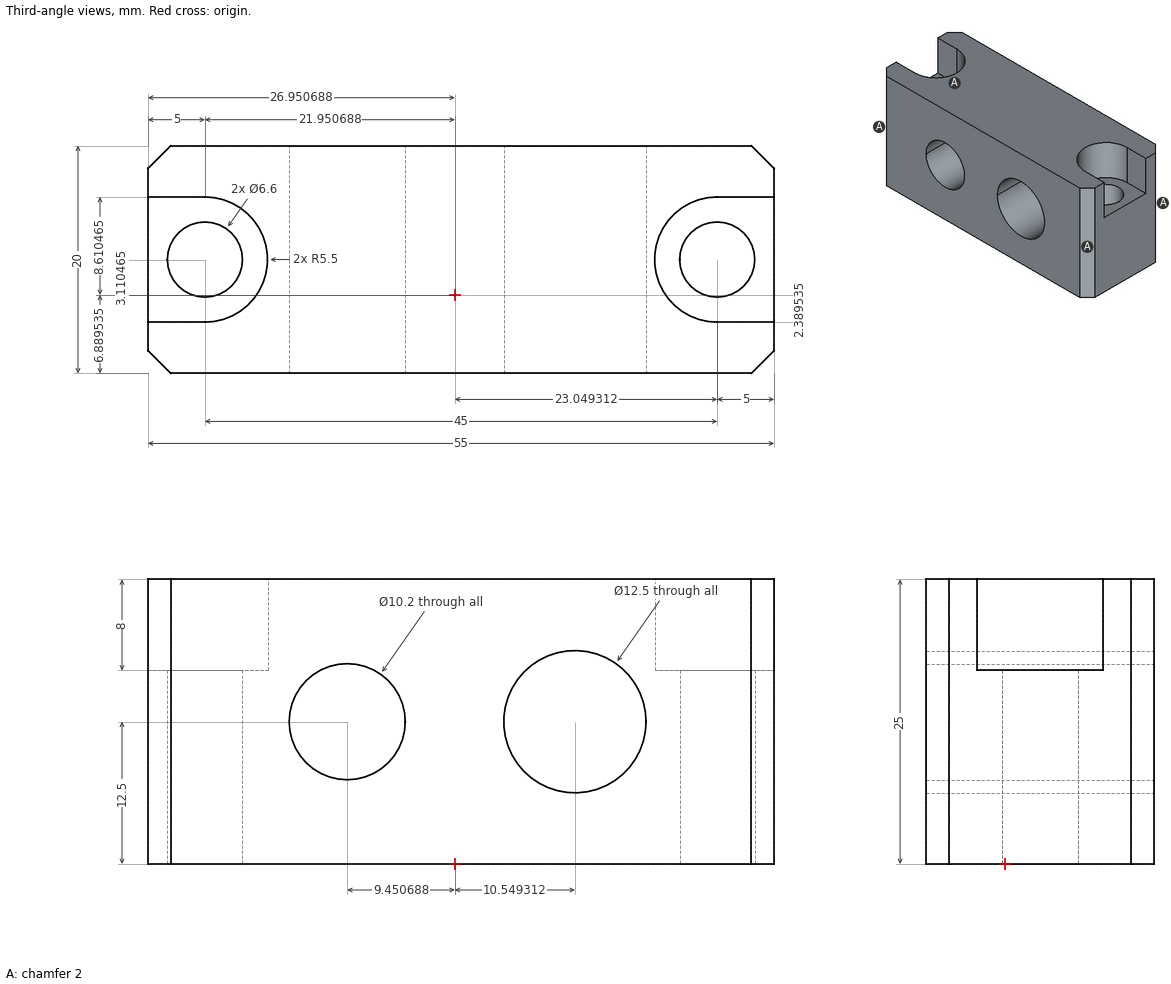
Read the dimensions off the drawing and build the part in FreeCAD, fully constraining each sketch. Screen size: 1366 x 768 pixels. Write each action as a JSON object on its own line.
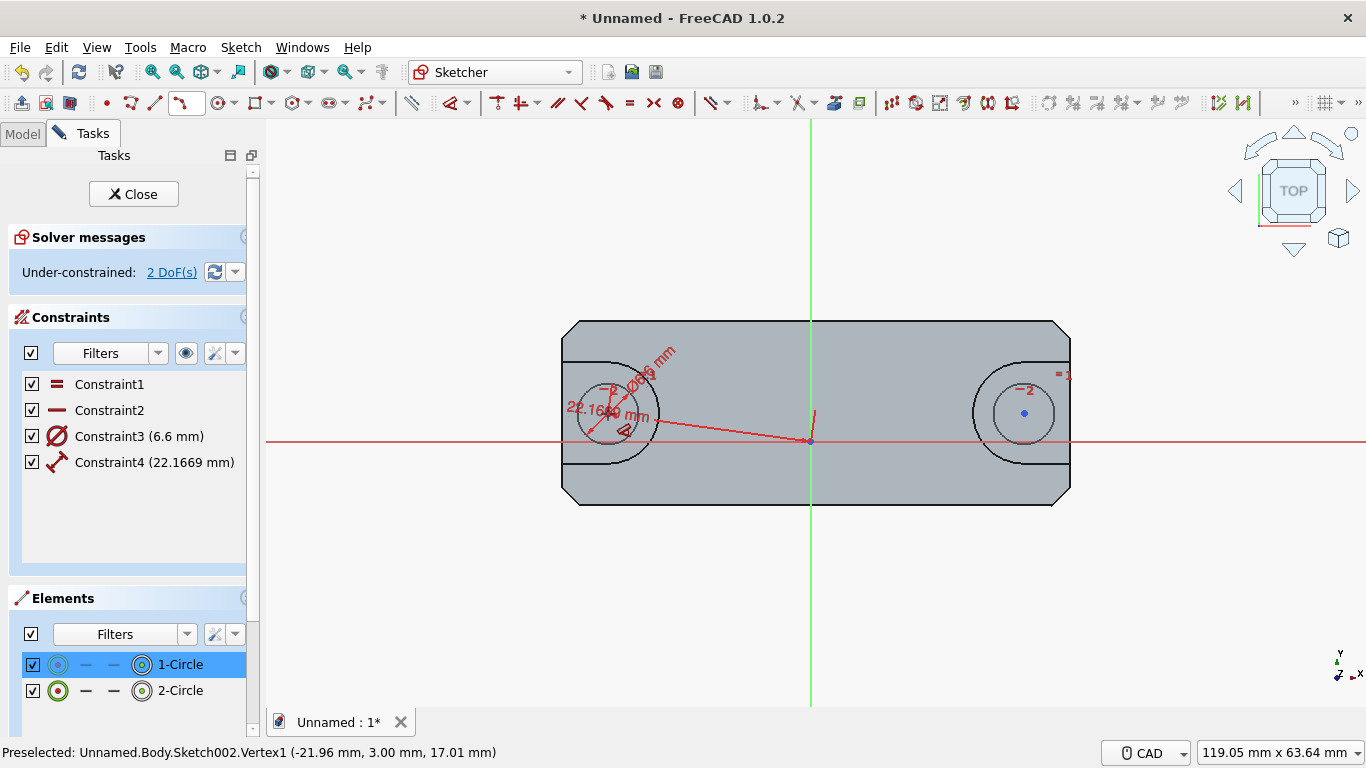
{"action": "left_click", "coordinate": [1024, 414]}
{"action": "left_click", "coordinate": [912, 380]}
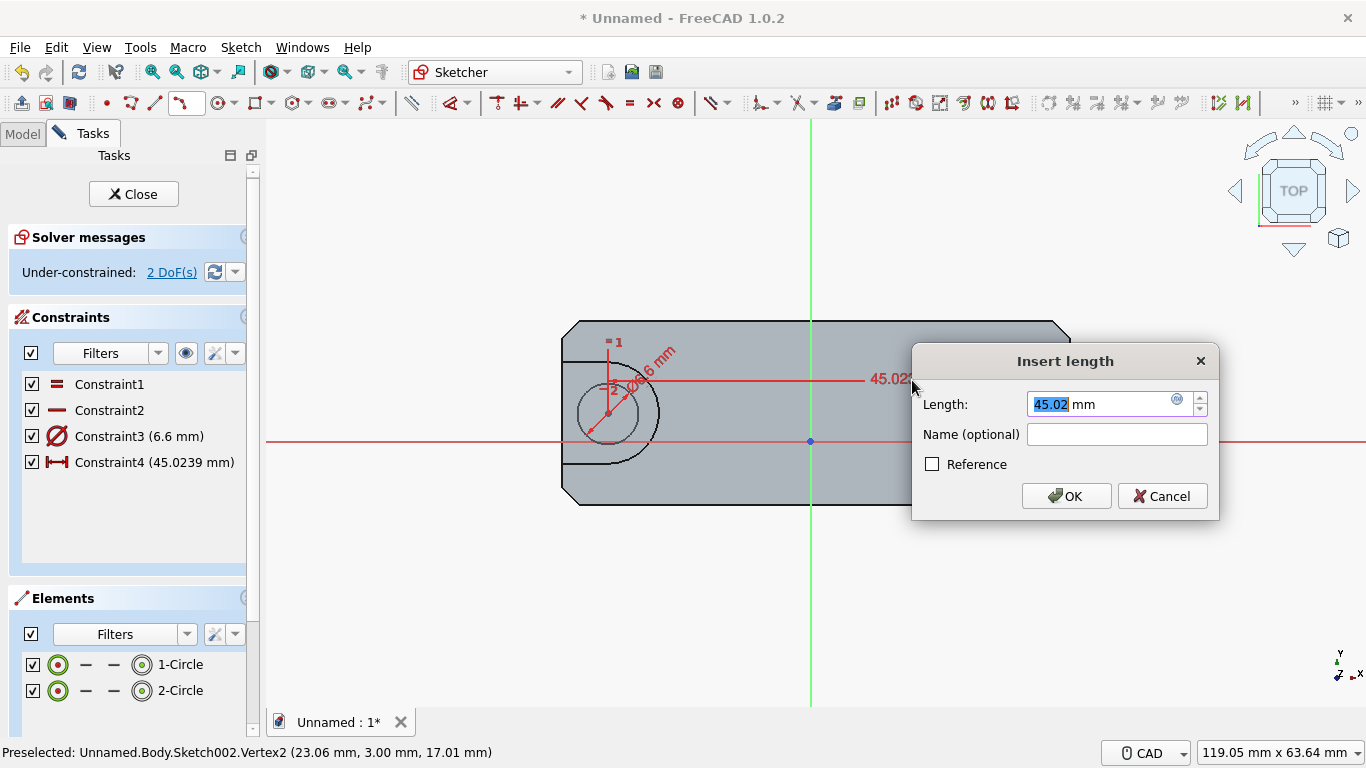
{"action": "type", "text": "45"}
{"action": "key", "text": "Return"}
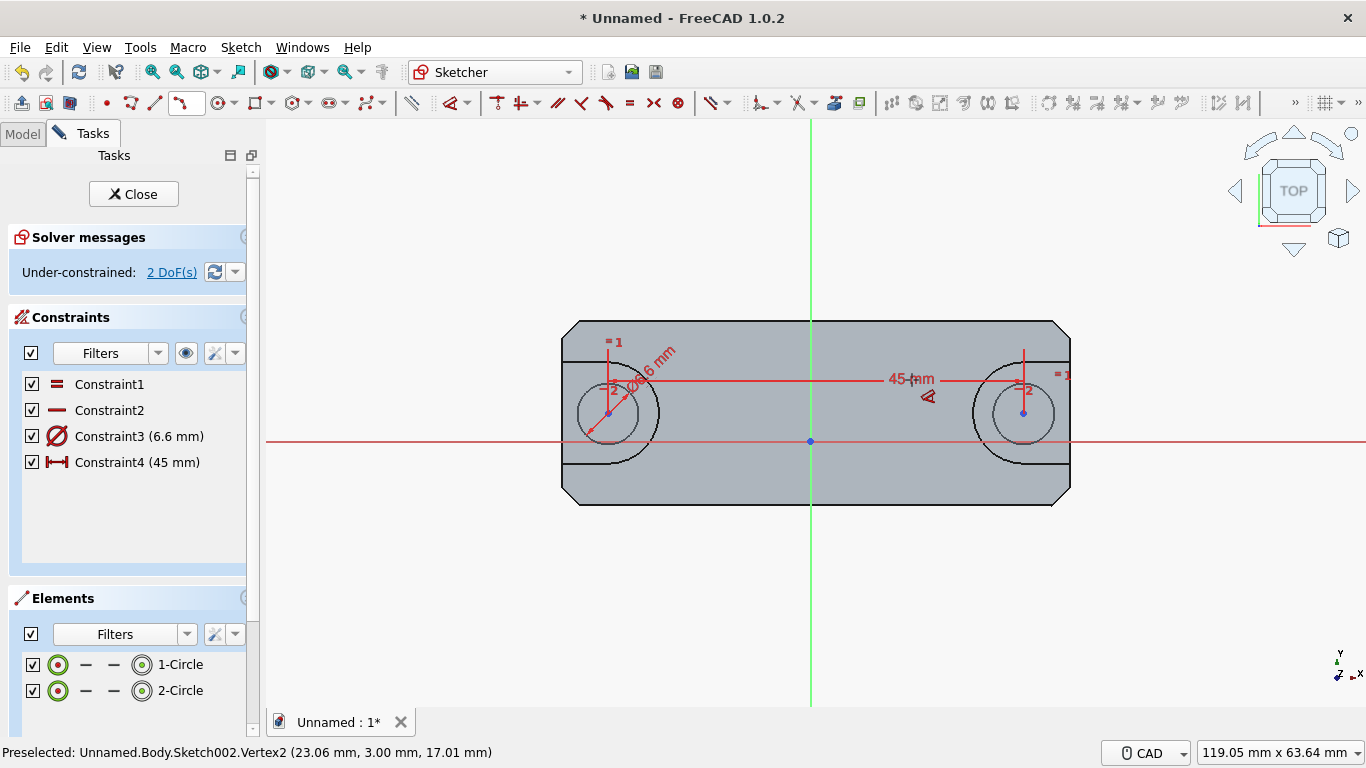
{"action": "scroll", "coordinate": [608, 414], "scroll_direction": "up", "scroll_amount": 2}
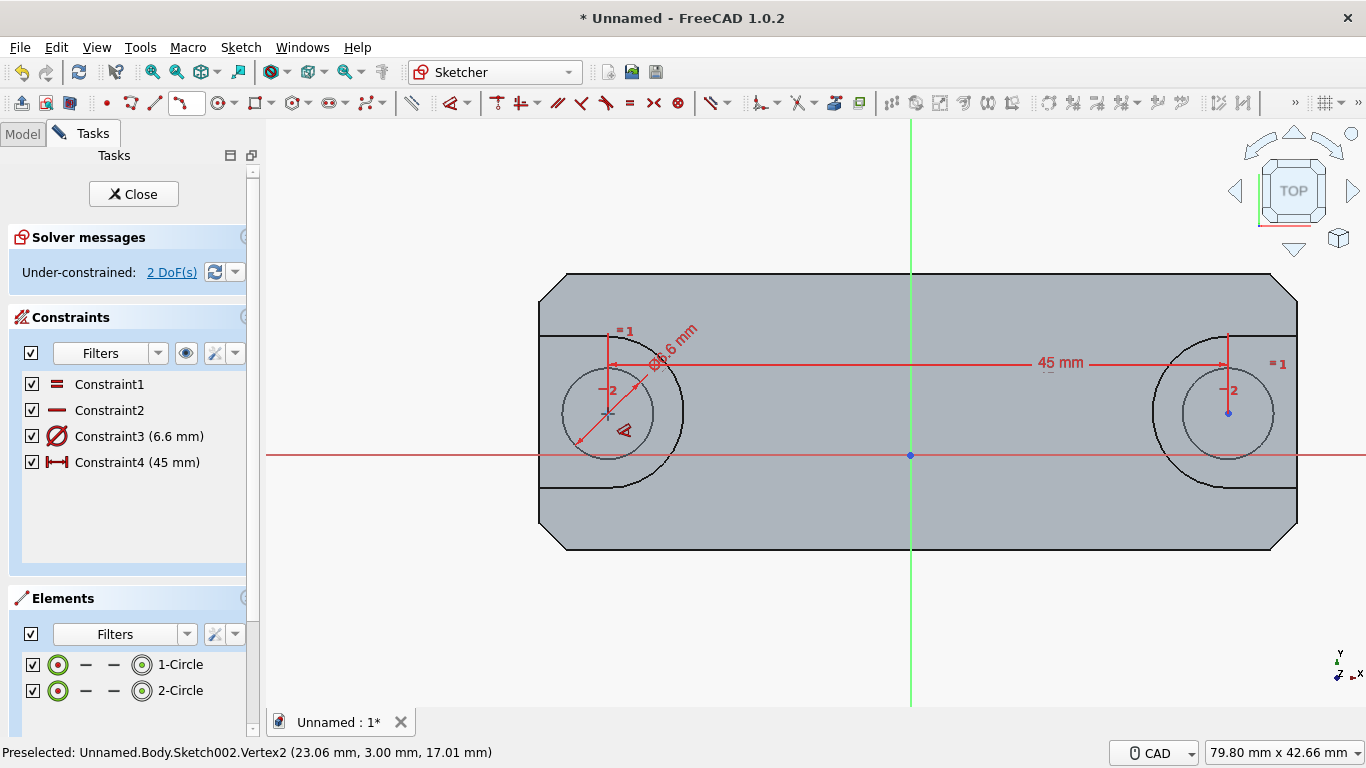
{"action": "left_click", "coordinate": [608, 414]}
{"action": "left_click", "coordinate": [945, 434]}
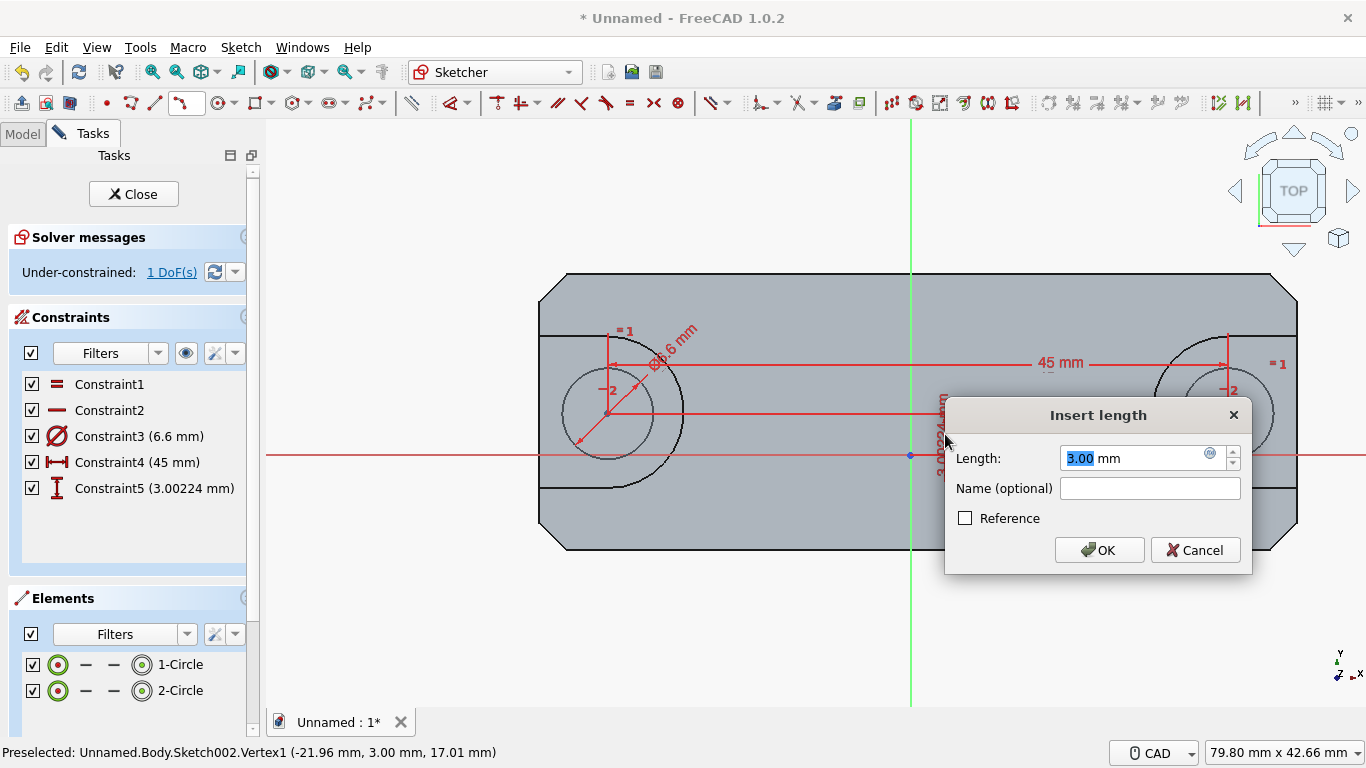
{"action": "type", "text": "3.110465"}
{"action": "key", "text": "Return"}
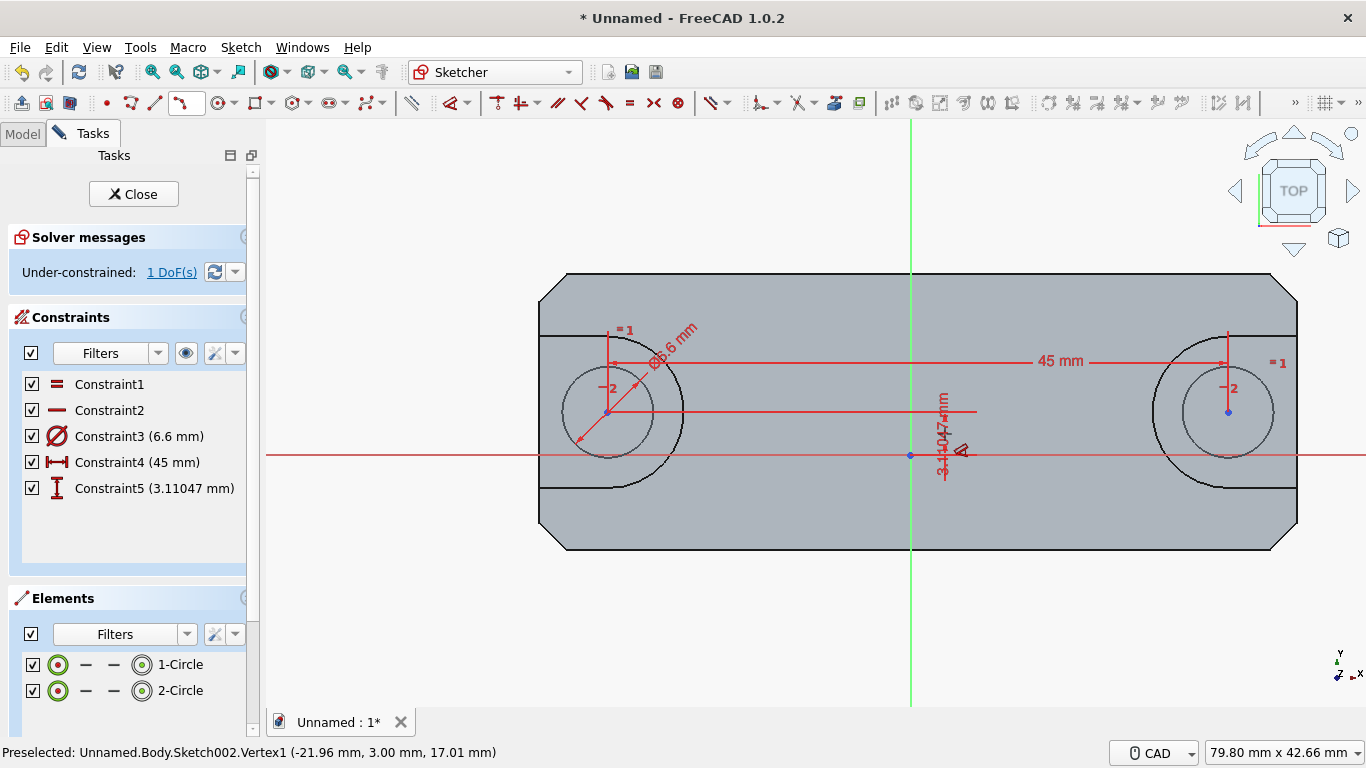
{"action": "left_click", "coordinate": [608, 412]}
{"action": "left_click", "coordinate": [759, 489]}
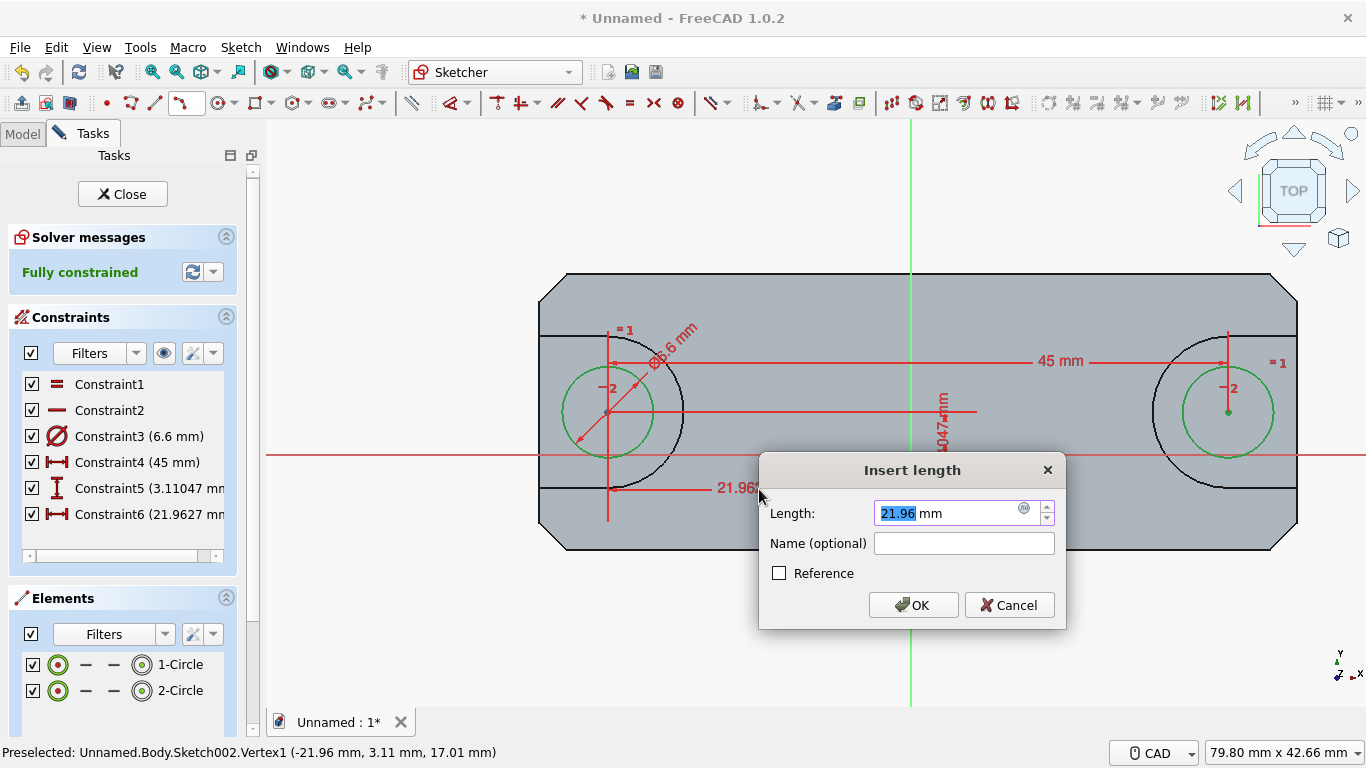
{"action": "type", "text": "21.950688"}
{"action": "key", "text": "Return"}
{"action": "key", "text": "Escape"}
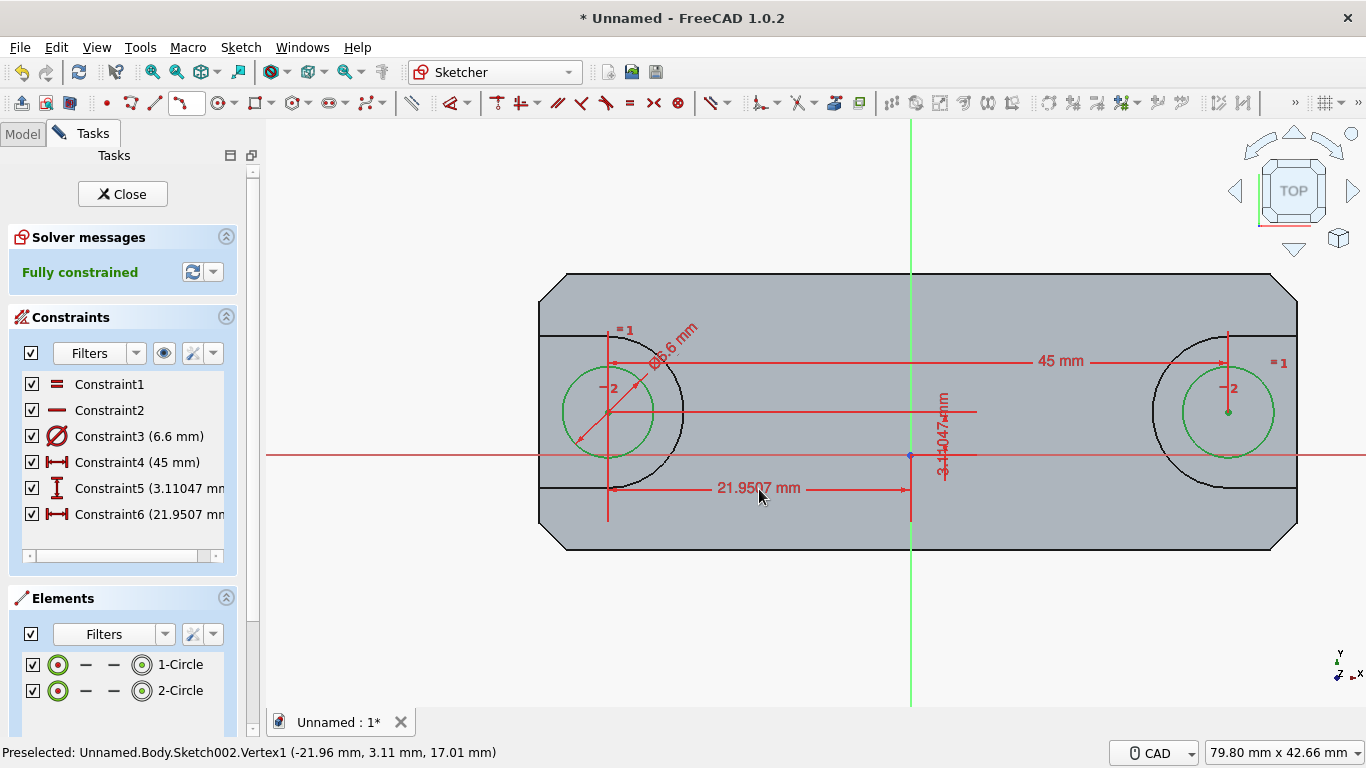
{"action": "left_click", "coordinate": [123, 194]}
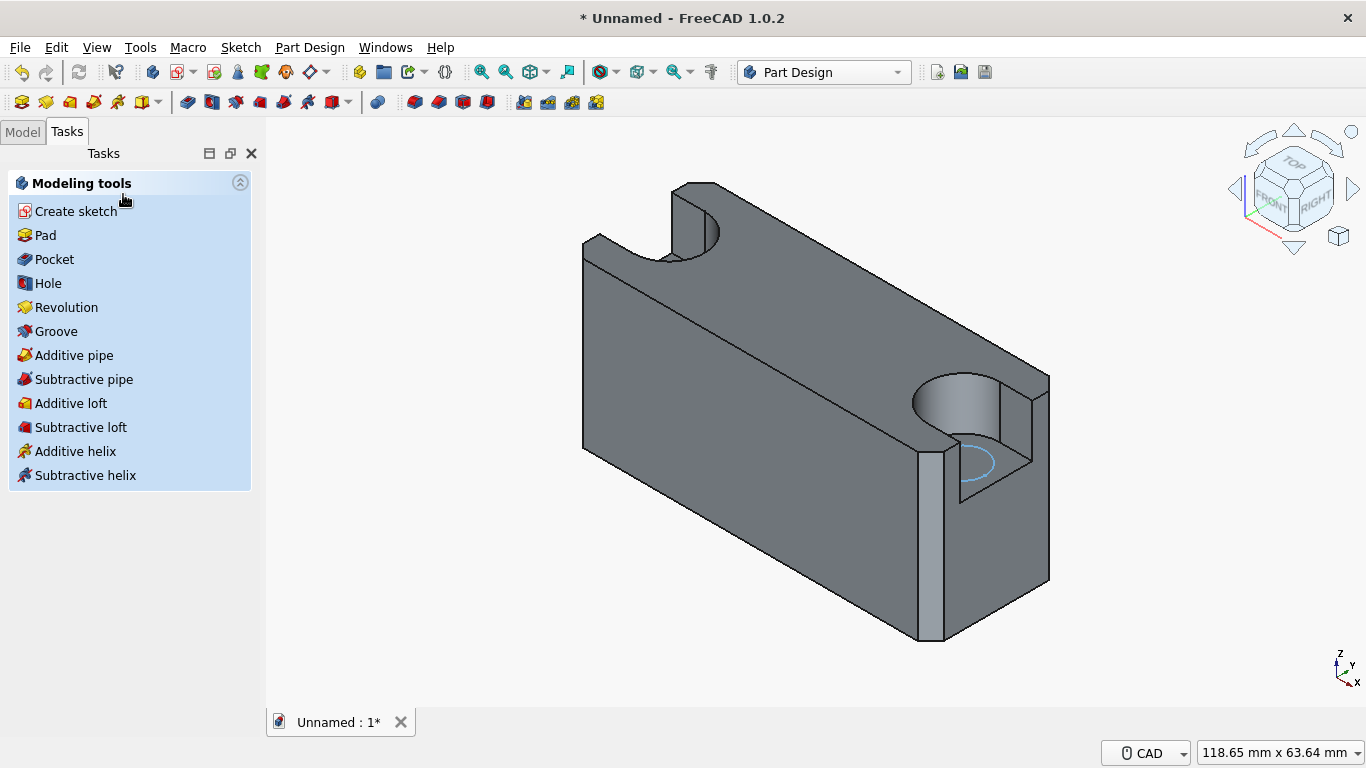
{"action": "left_click", "coordinate": [188, 102]}